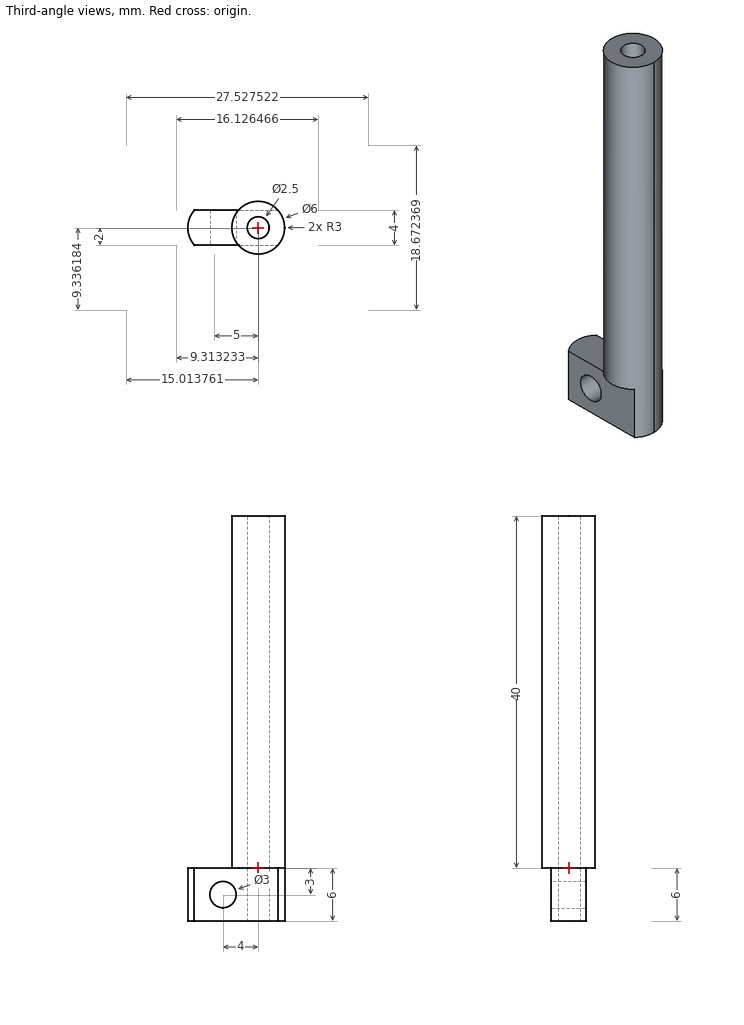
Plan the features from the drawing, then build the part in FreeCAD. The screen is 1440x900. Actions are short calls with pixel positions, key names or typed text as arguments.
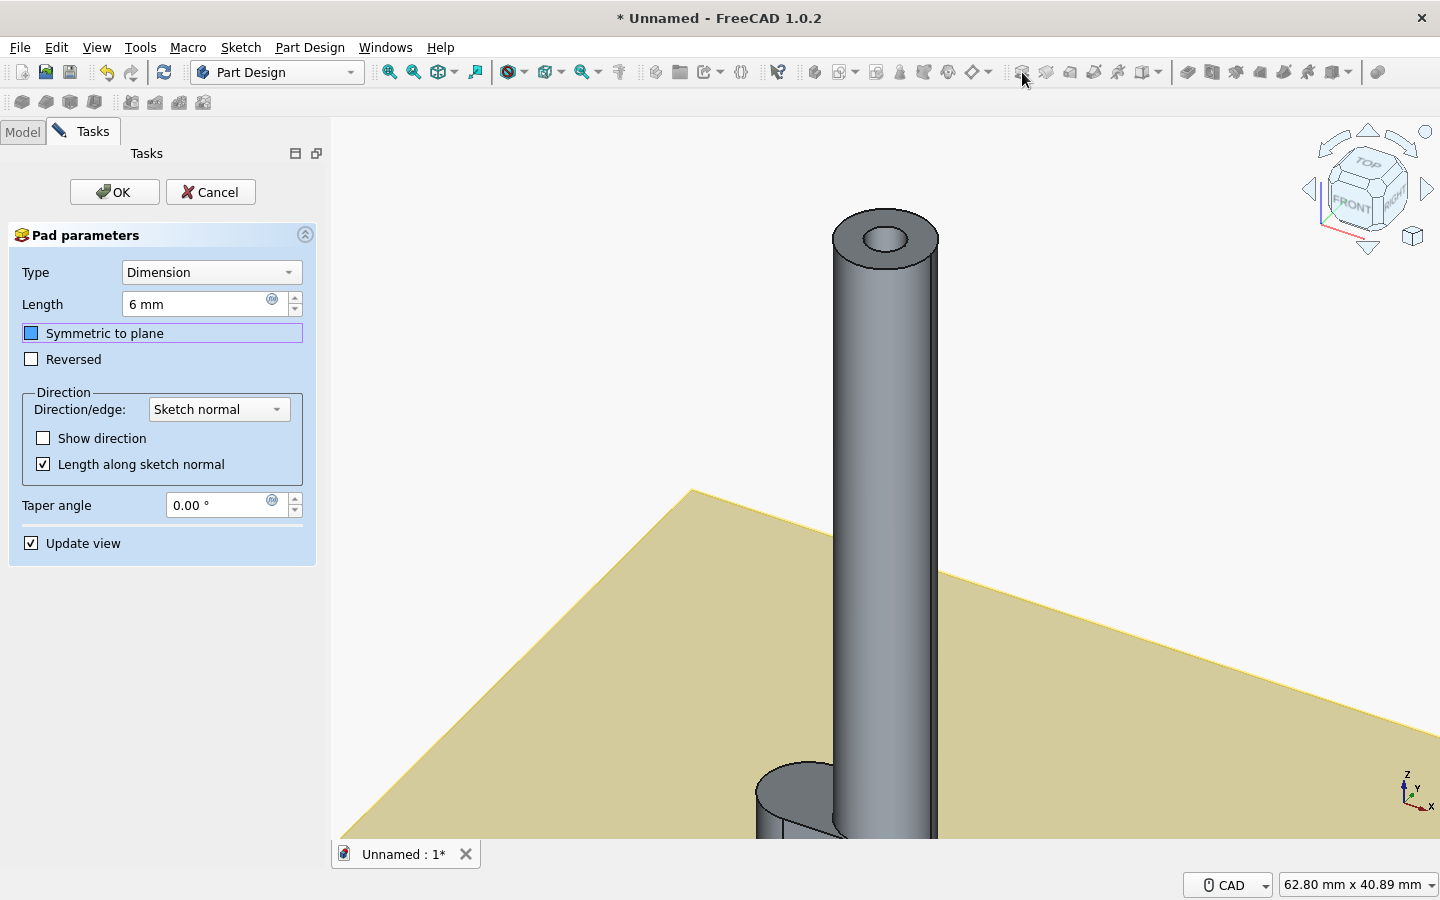
click(115, 192)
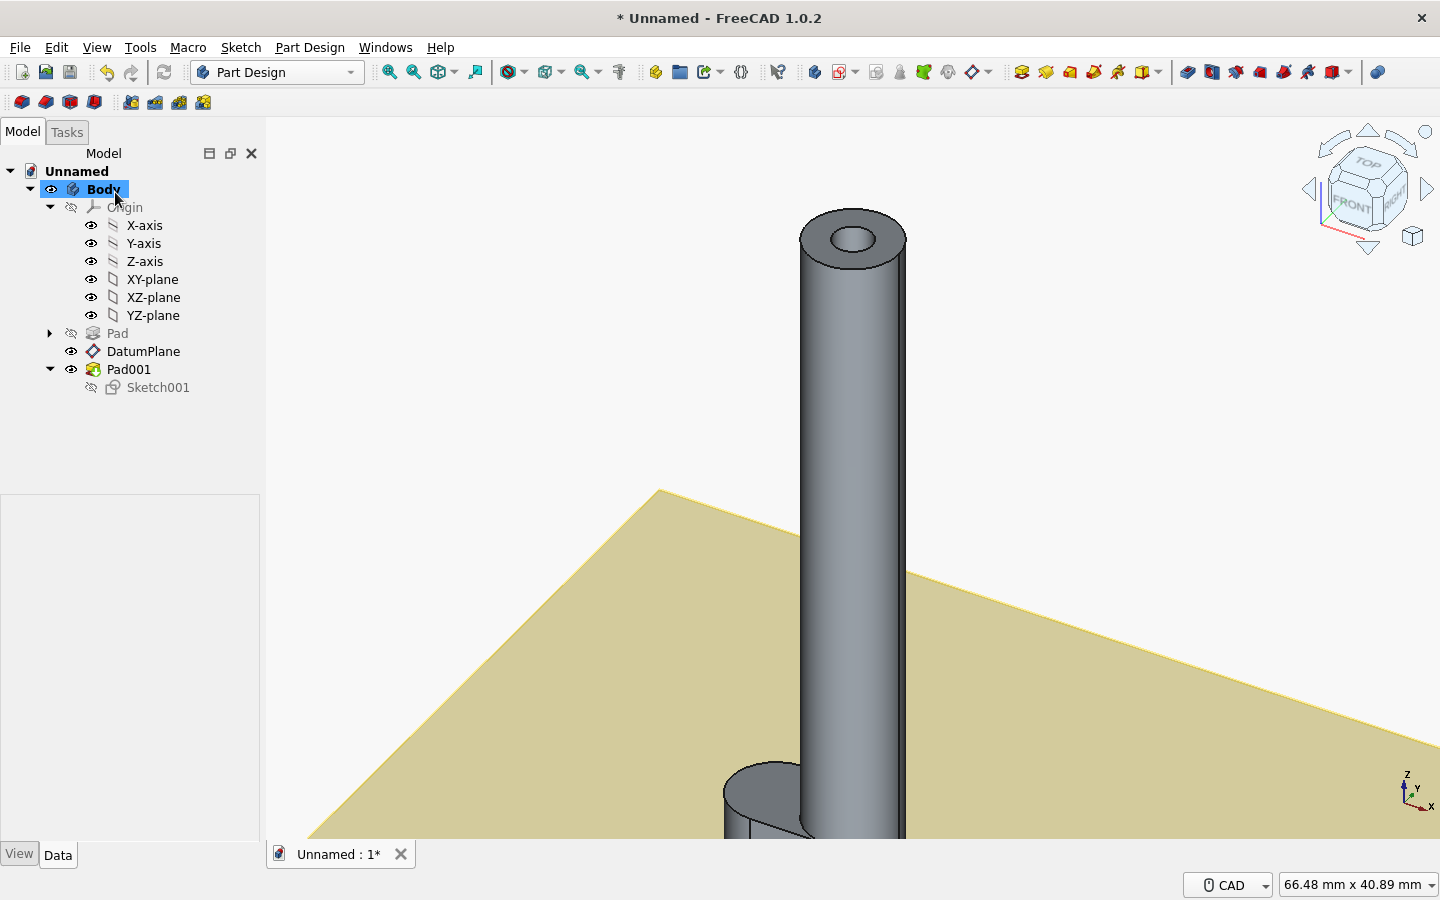
click(116, 351)
key(space)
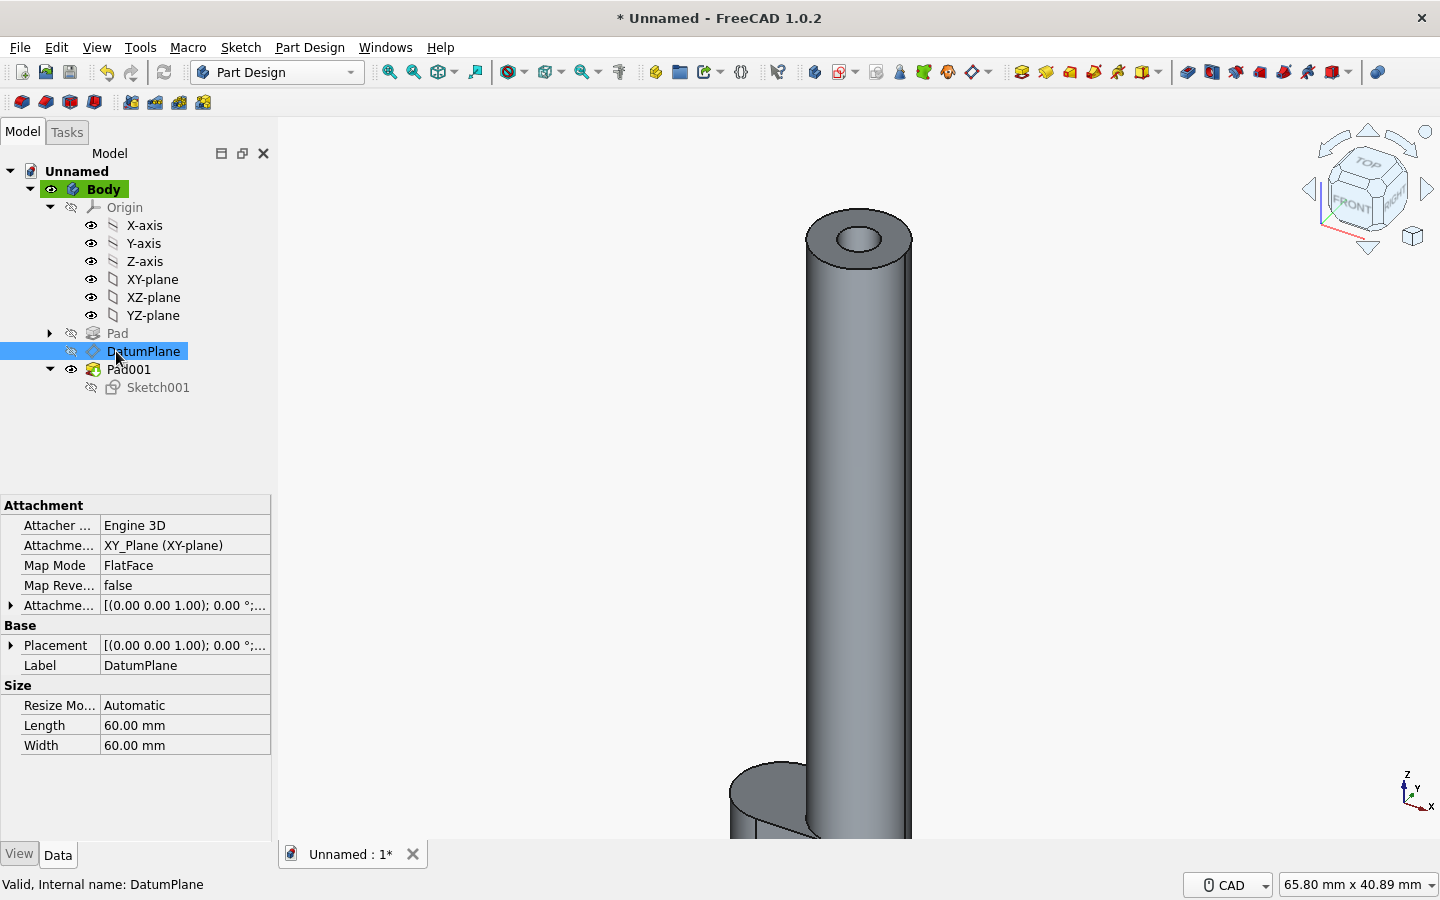
key(v)
key(f)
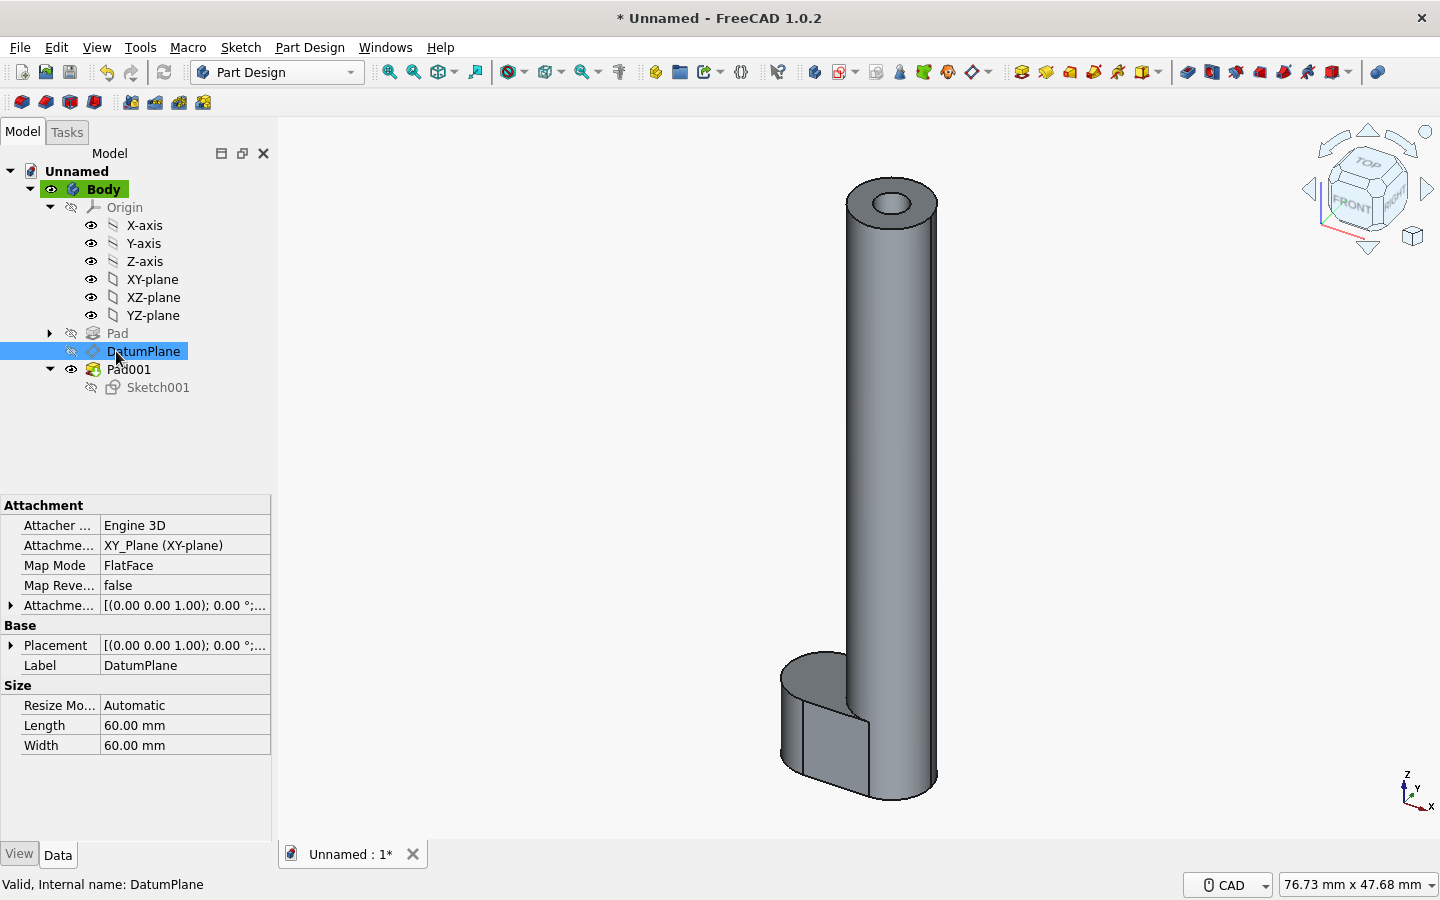
key(5)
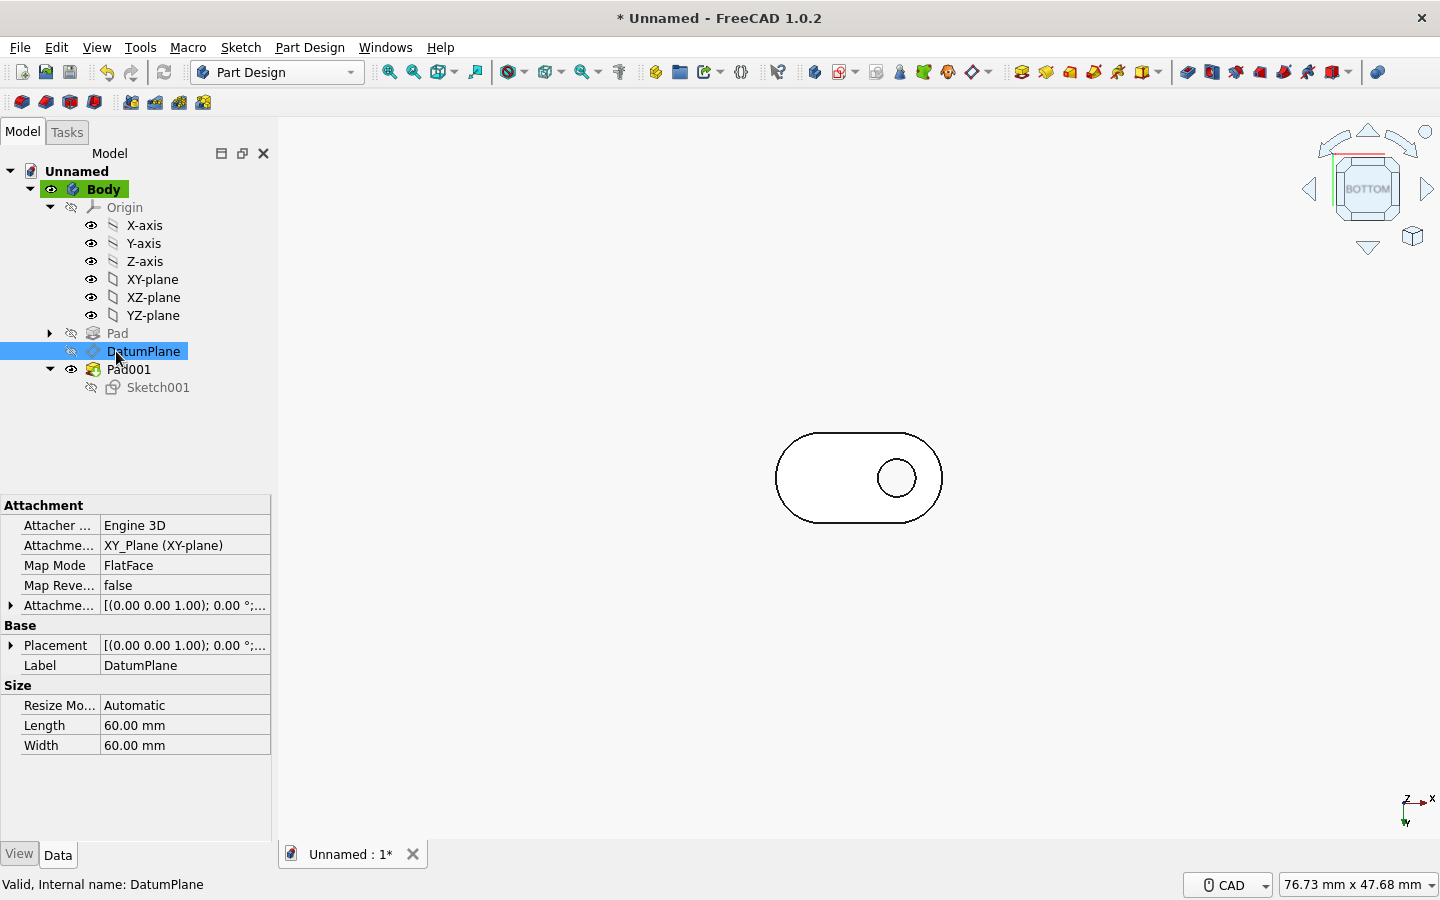
click(390, 72)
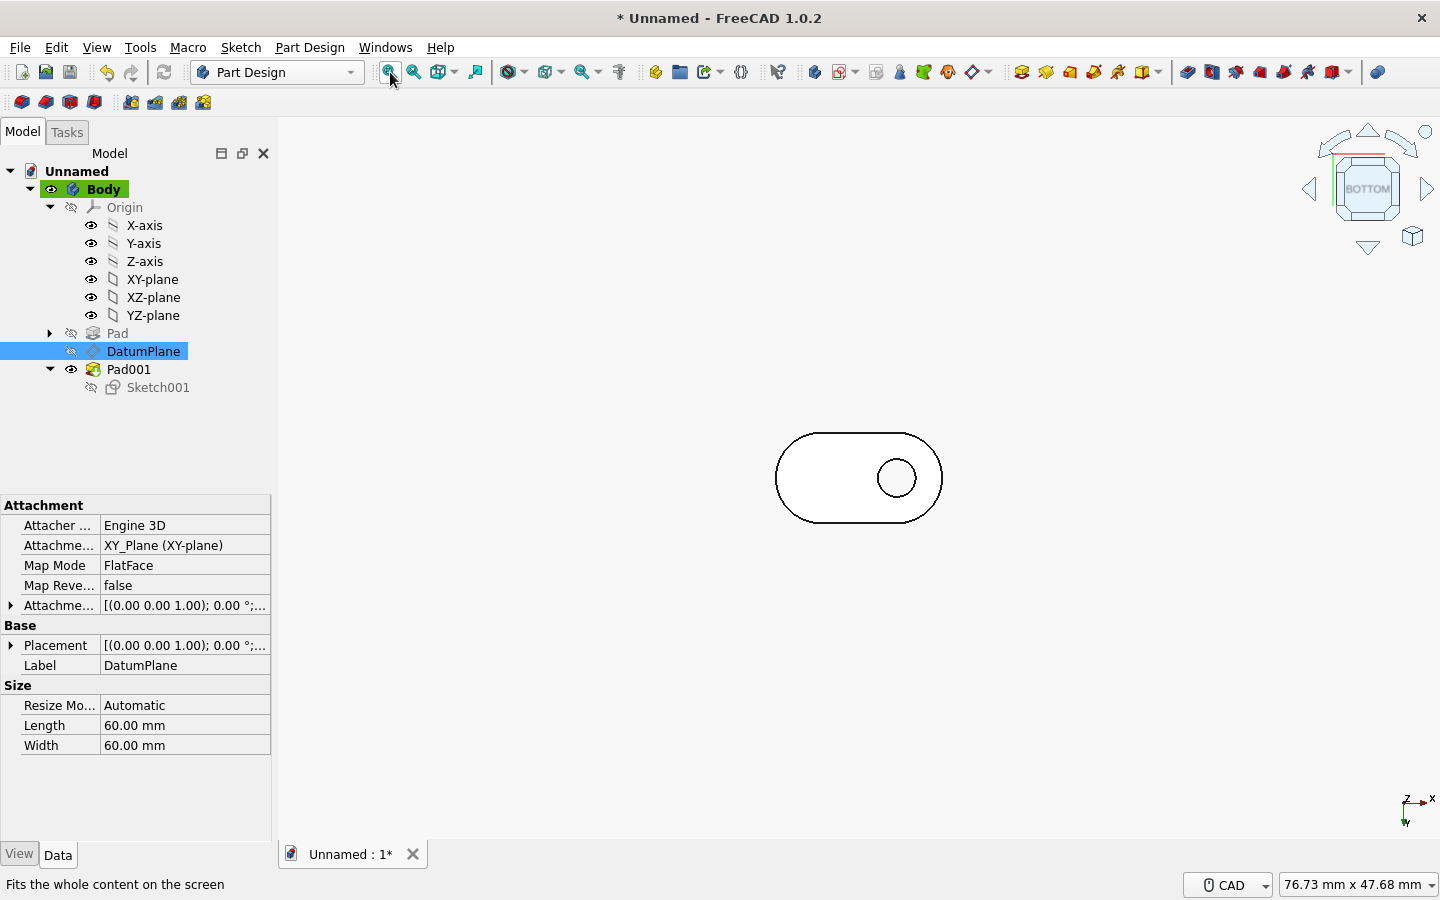
click(835, 477)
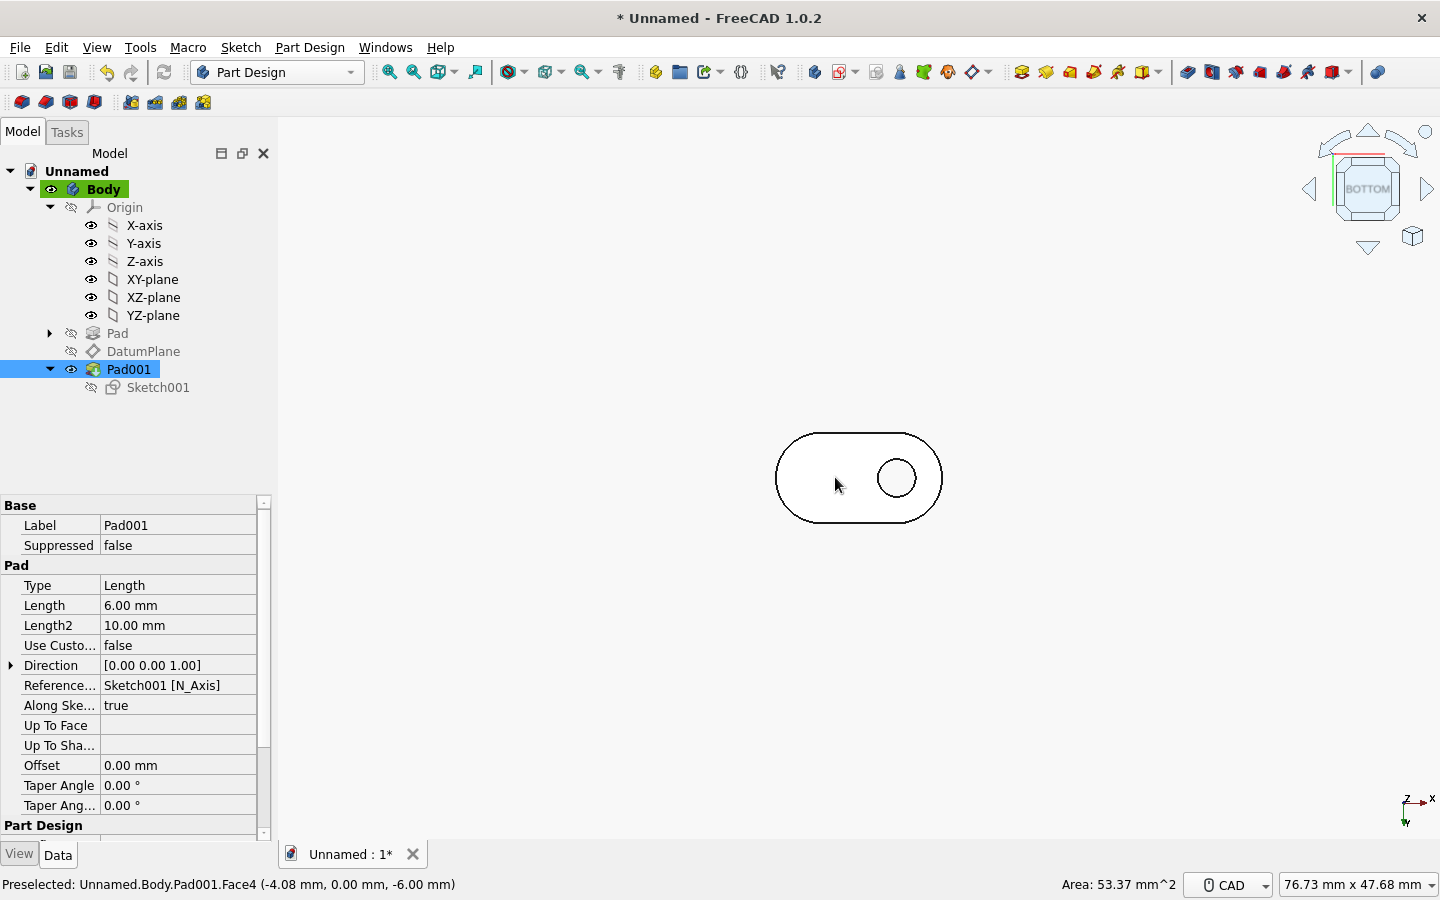
click(840, 72)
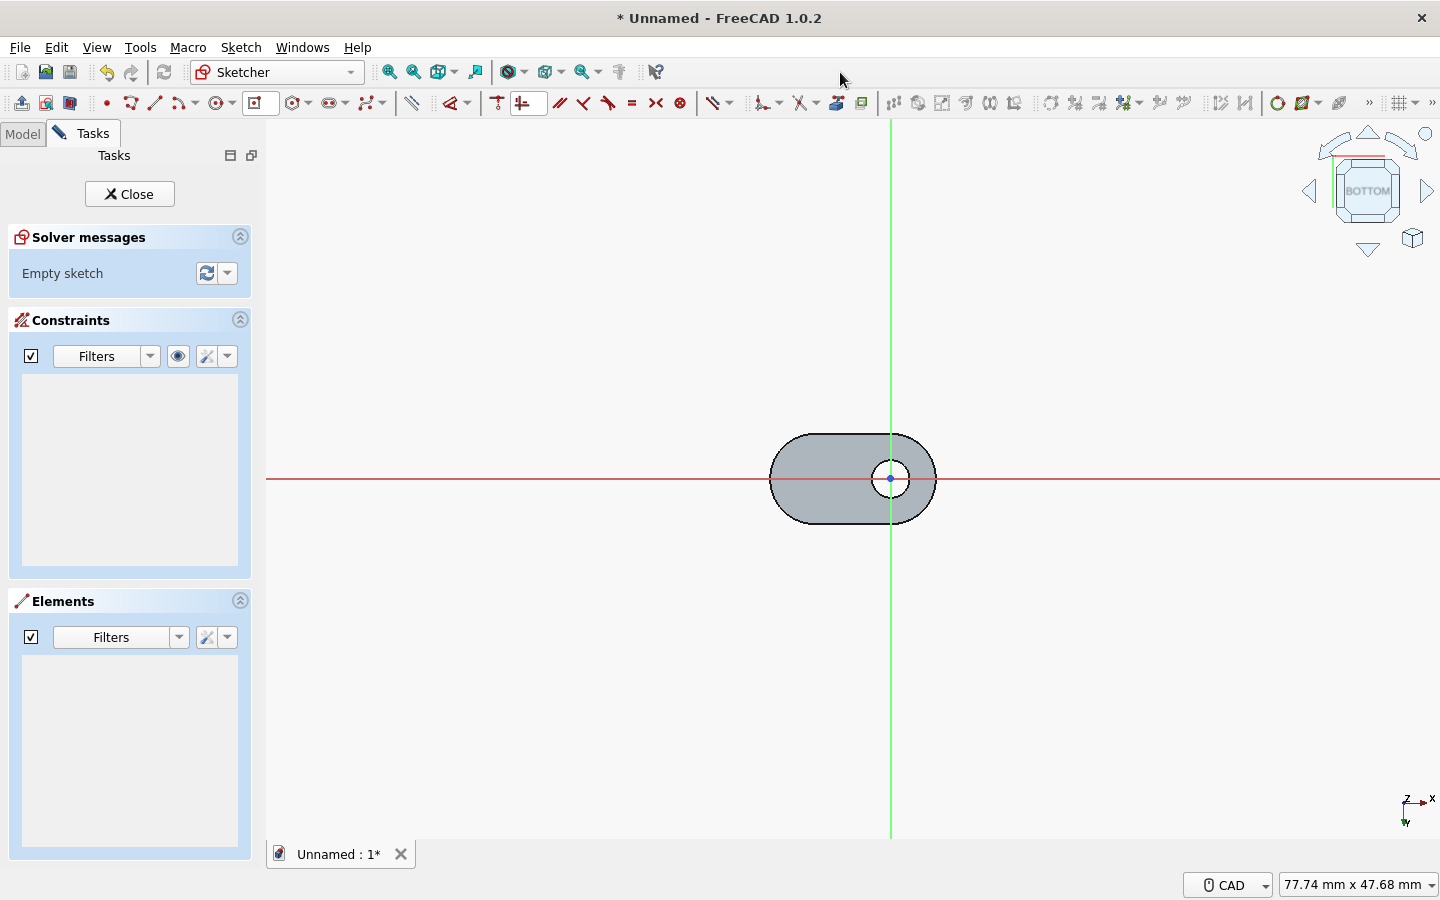
scroll(978, 479, up, 3)